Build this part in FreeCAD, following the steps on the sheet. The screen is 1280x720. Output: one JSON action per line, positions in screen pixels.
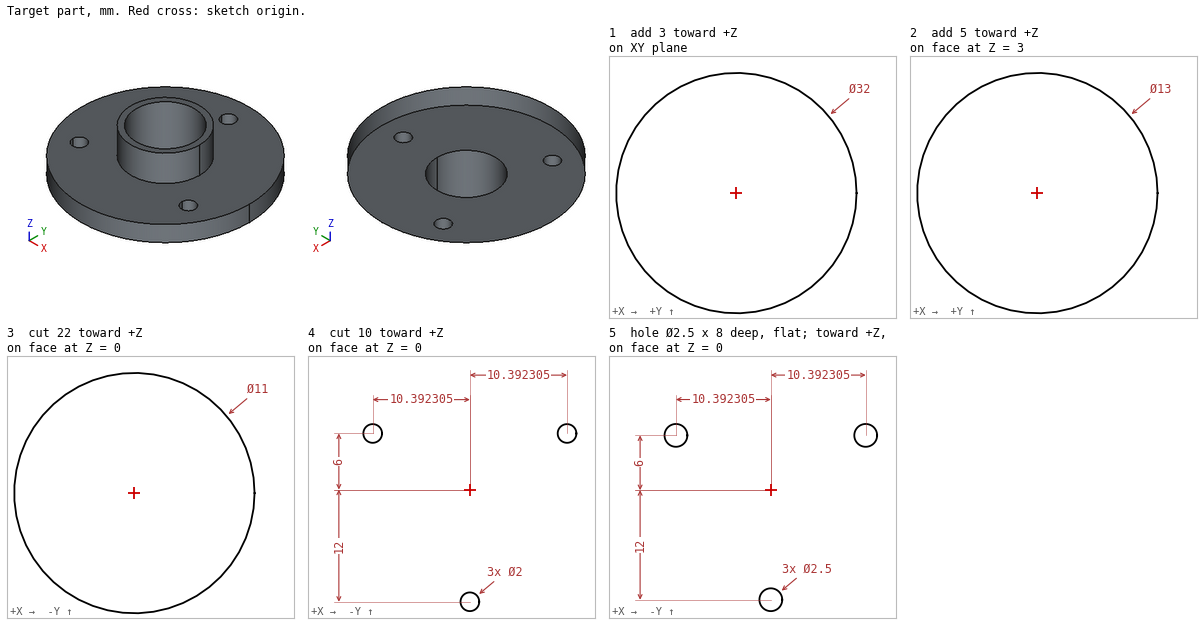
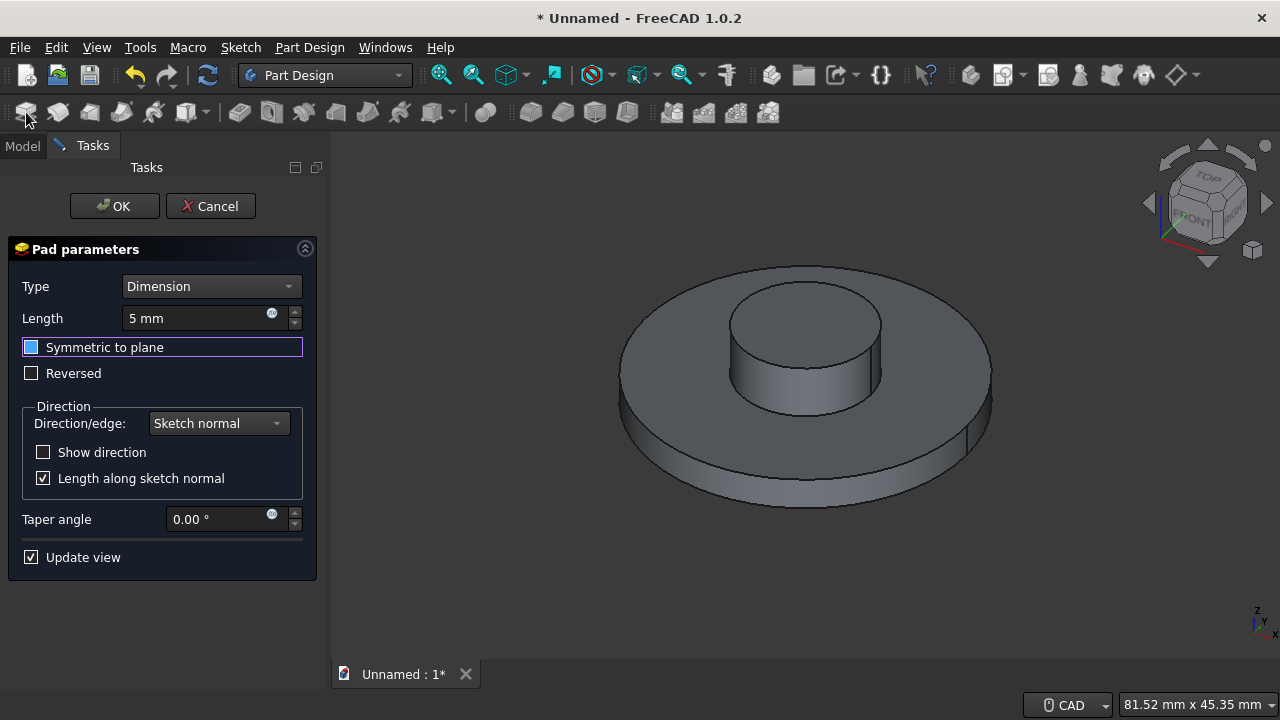
{"action": "left_click", "coordinate": [115, 206]}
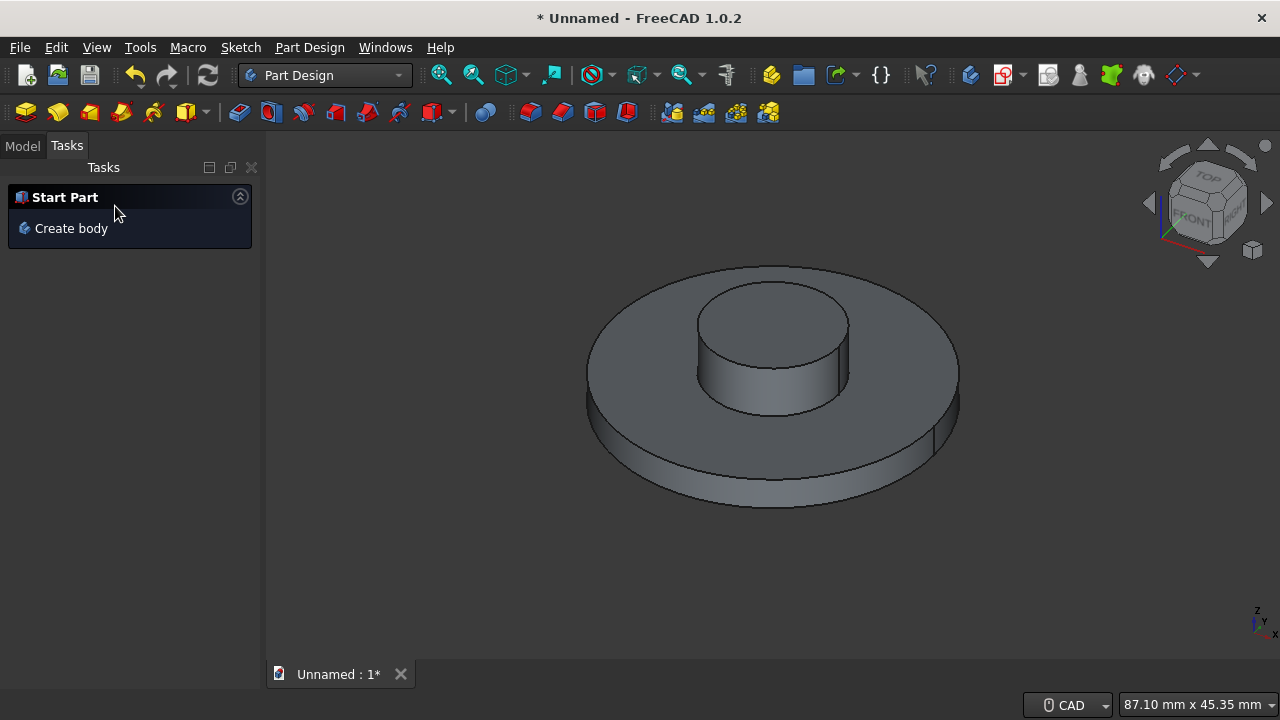
{"action": "key", "text": "5"}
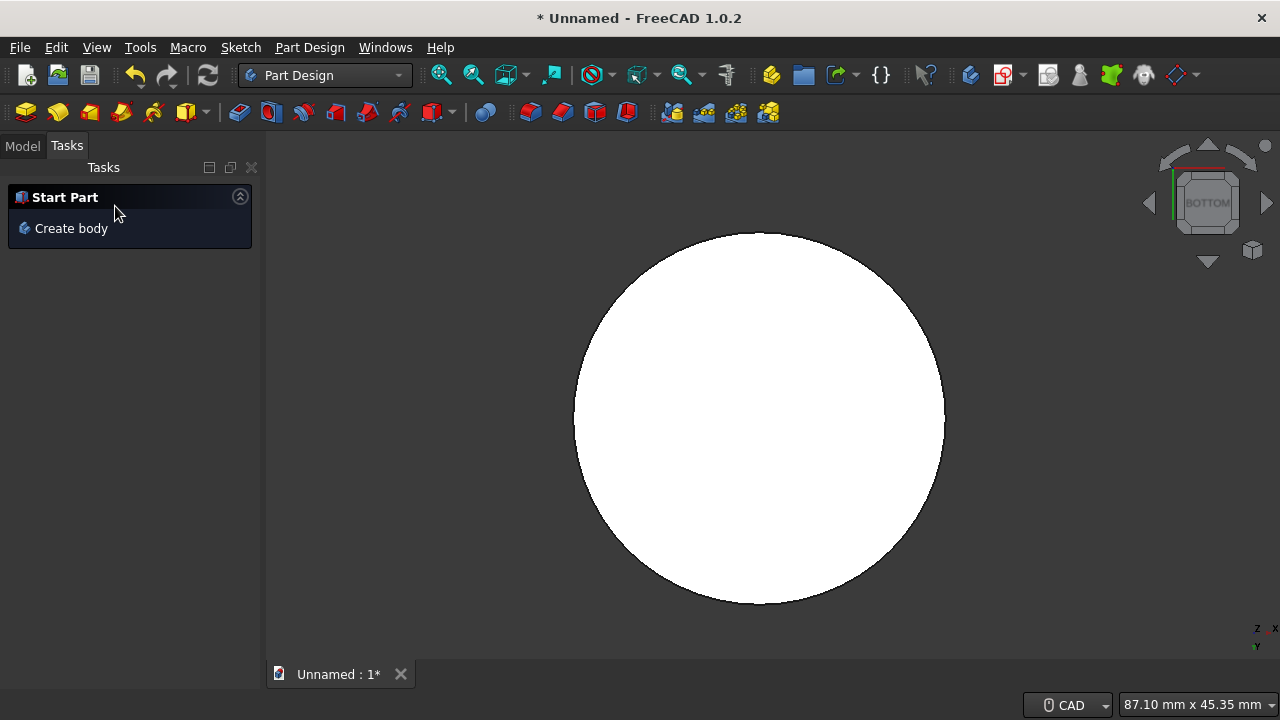
{"action": "left_click", "coordinate": [759, 418]}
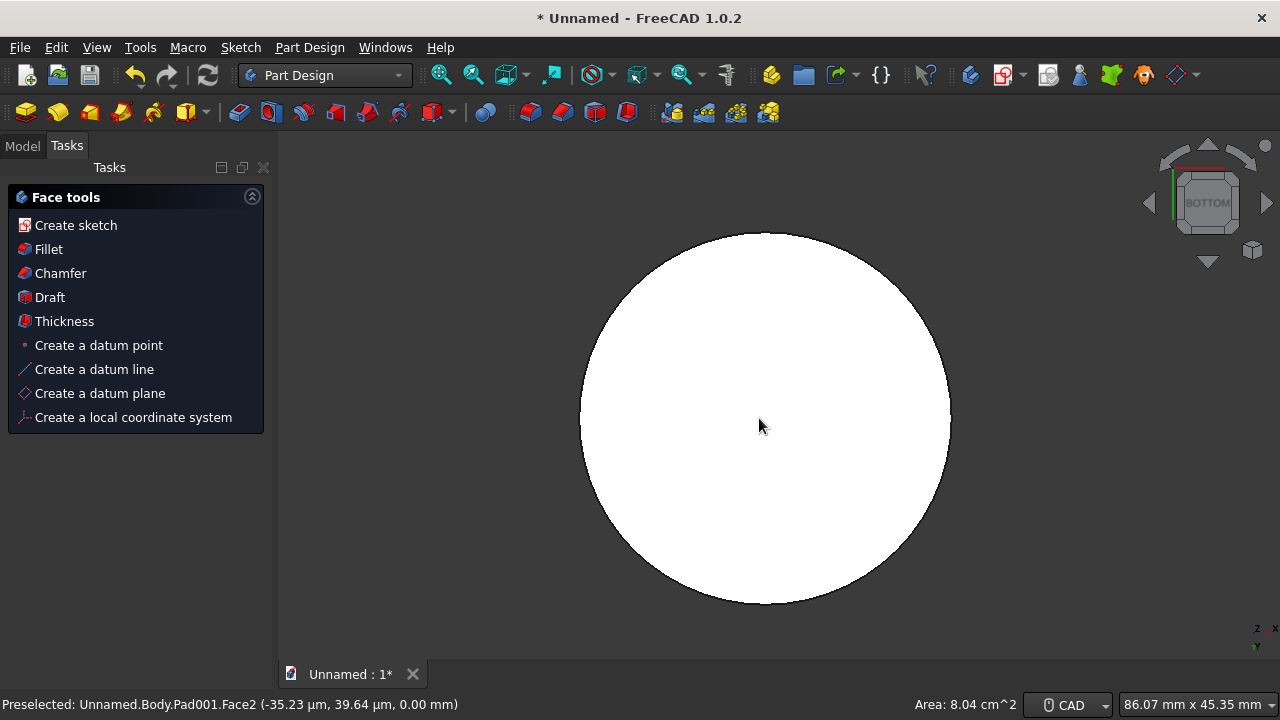
{"action": "left_click", "coordinate": [1004, 76]}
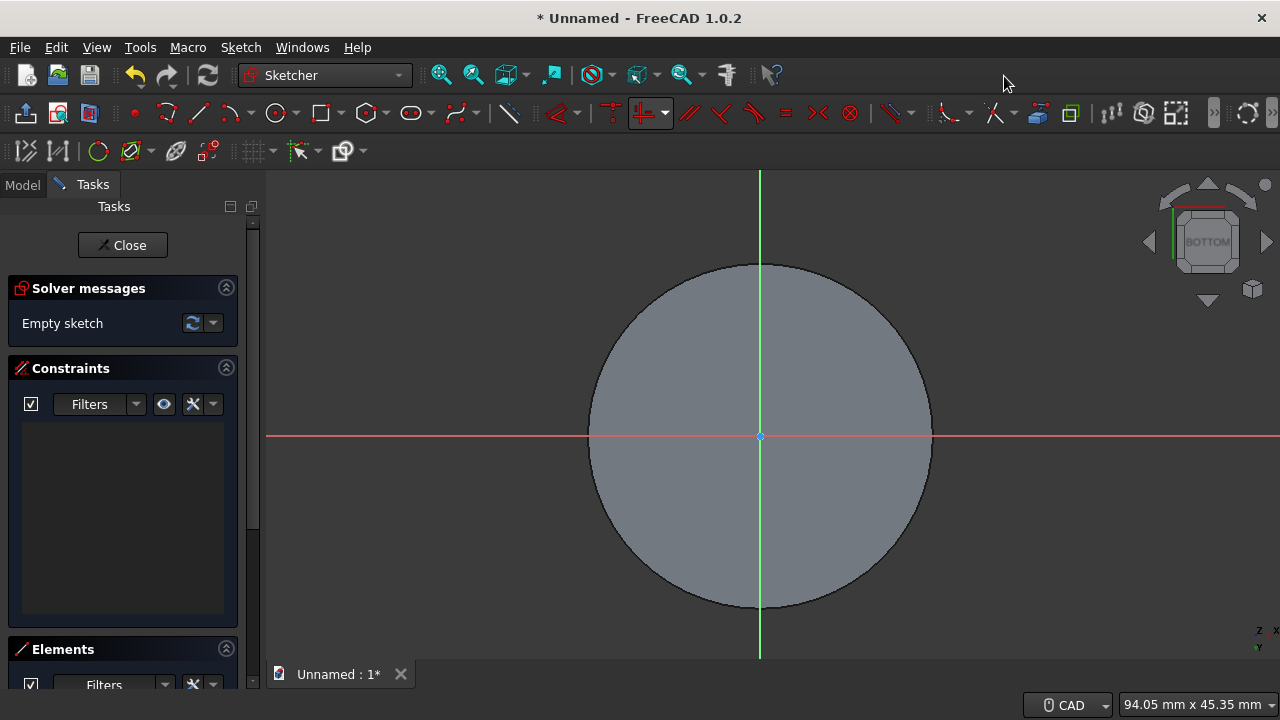
{"action": "scroll", "coordinate": [793, 449], "scroll_direction": "up", "scroll_amount": 5}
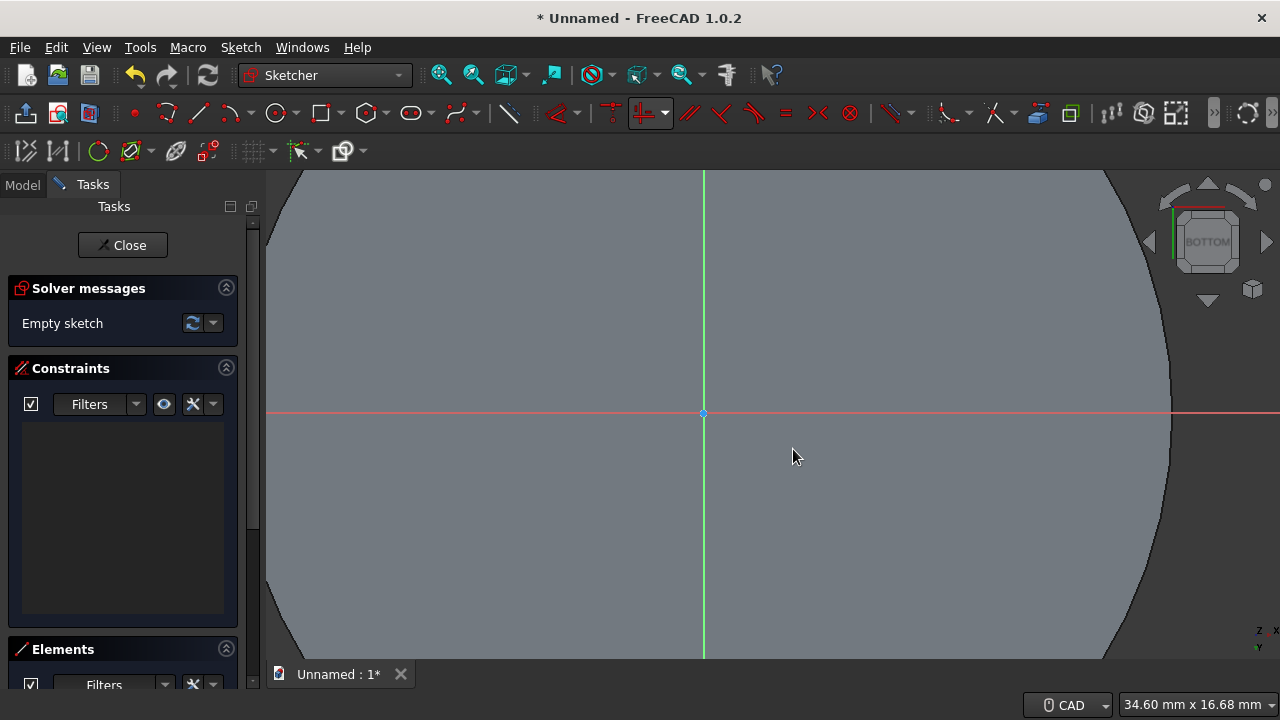
{"action": "left_click", "coordinate": [276, 114]}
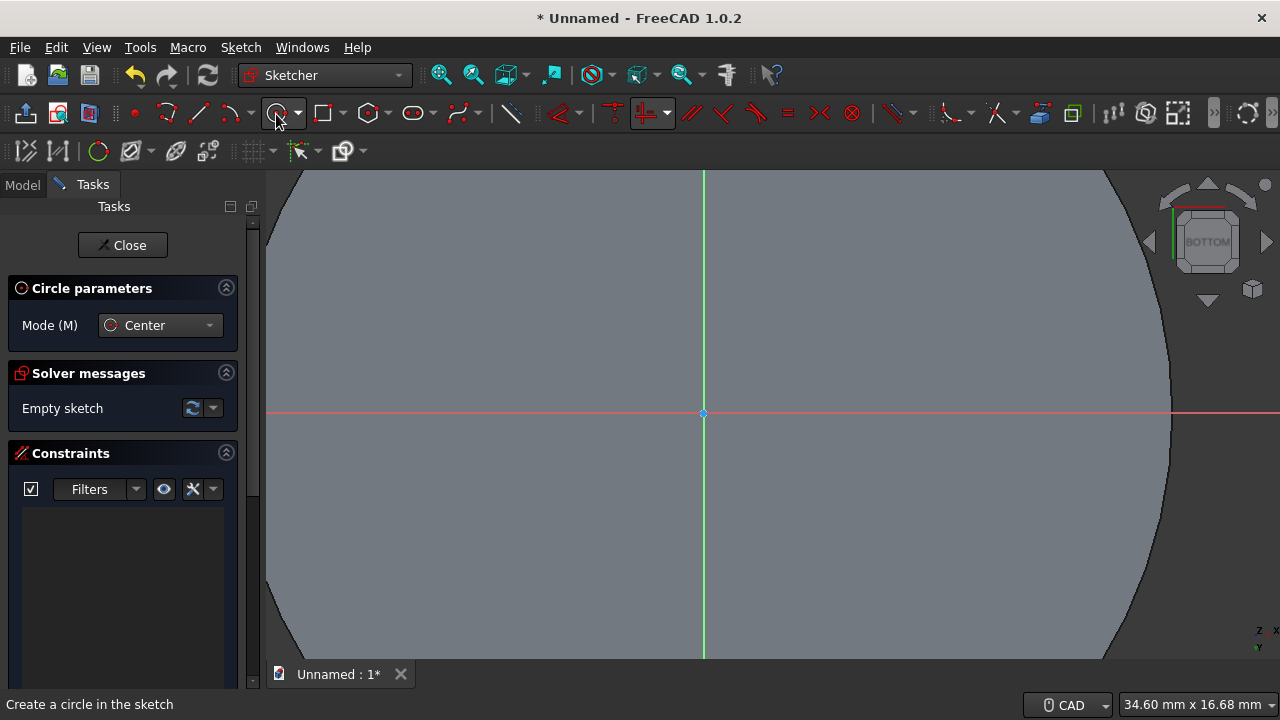
{"action": "left_click", "coordinate": [704, 413]}
{"action": "mouse_move", "coordinate": [818, 300]}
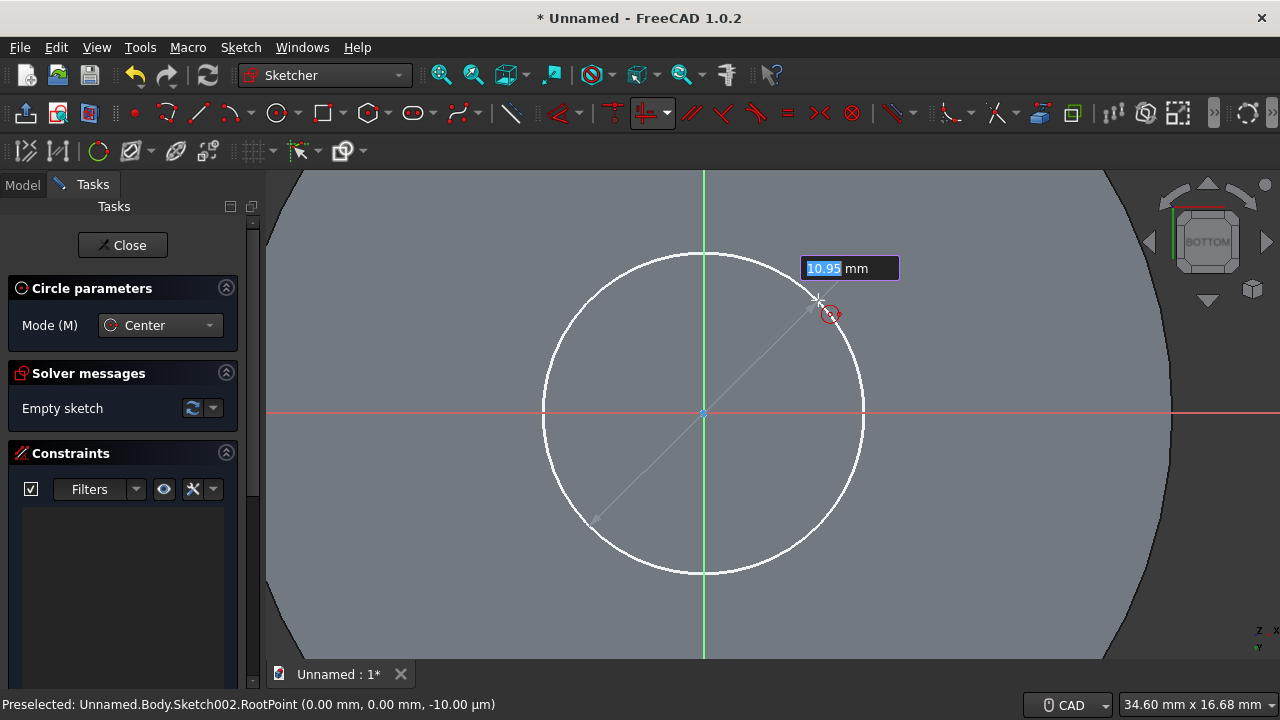
{"action": "type", "text": "11"}
{"action": "key", "text": "Return"}
{"action": "key", "text": "Escape"}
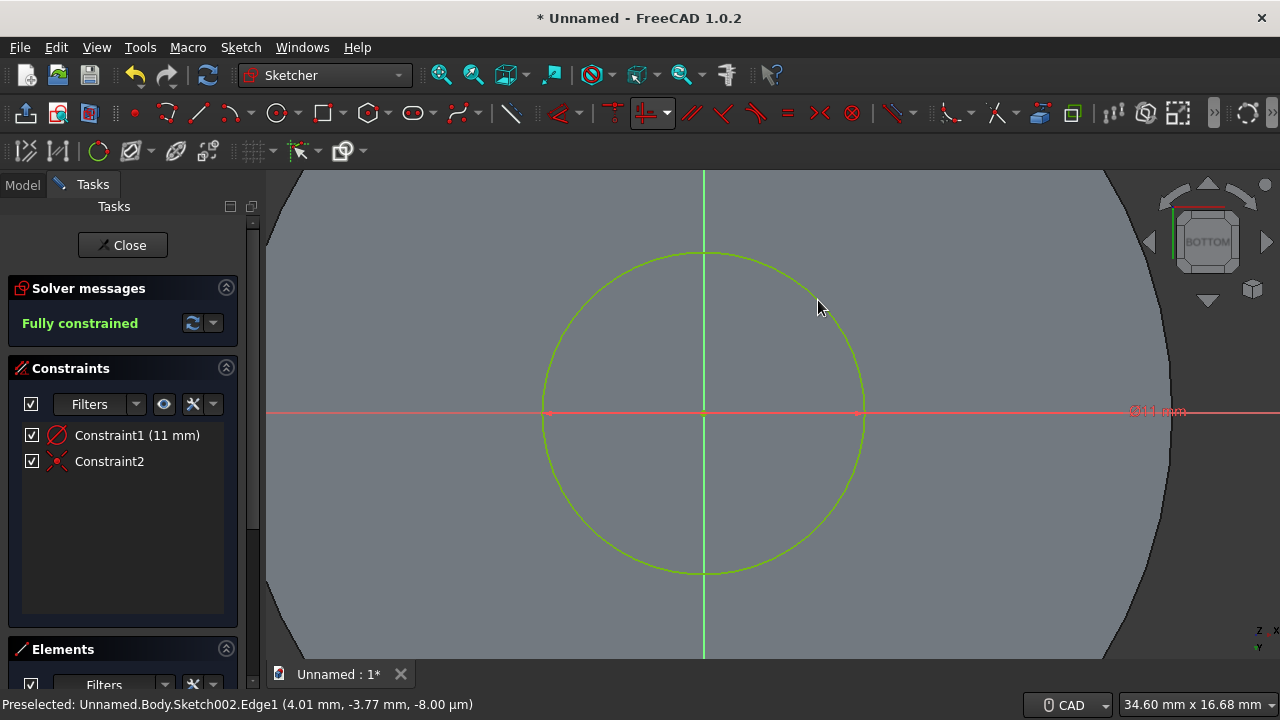
{"action": "left_click", "coordinate": [123, 245]}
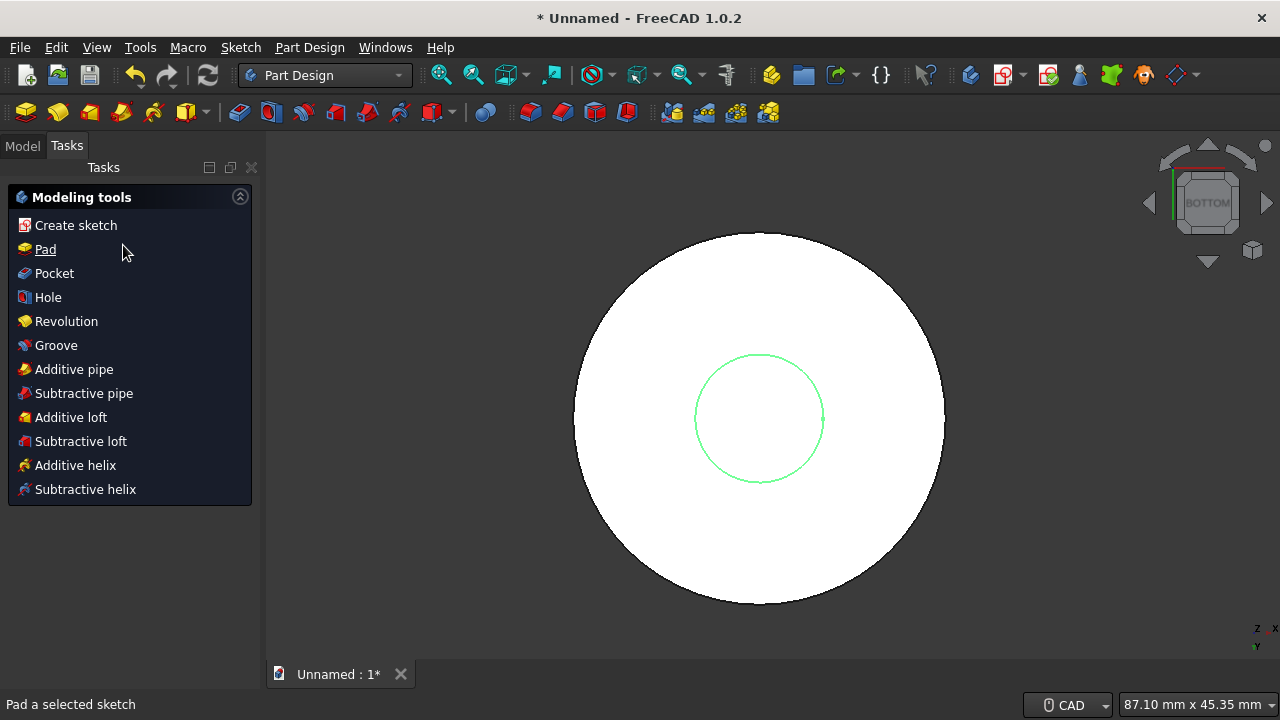
{"action": "left_click", "coordinate": [240, 112]}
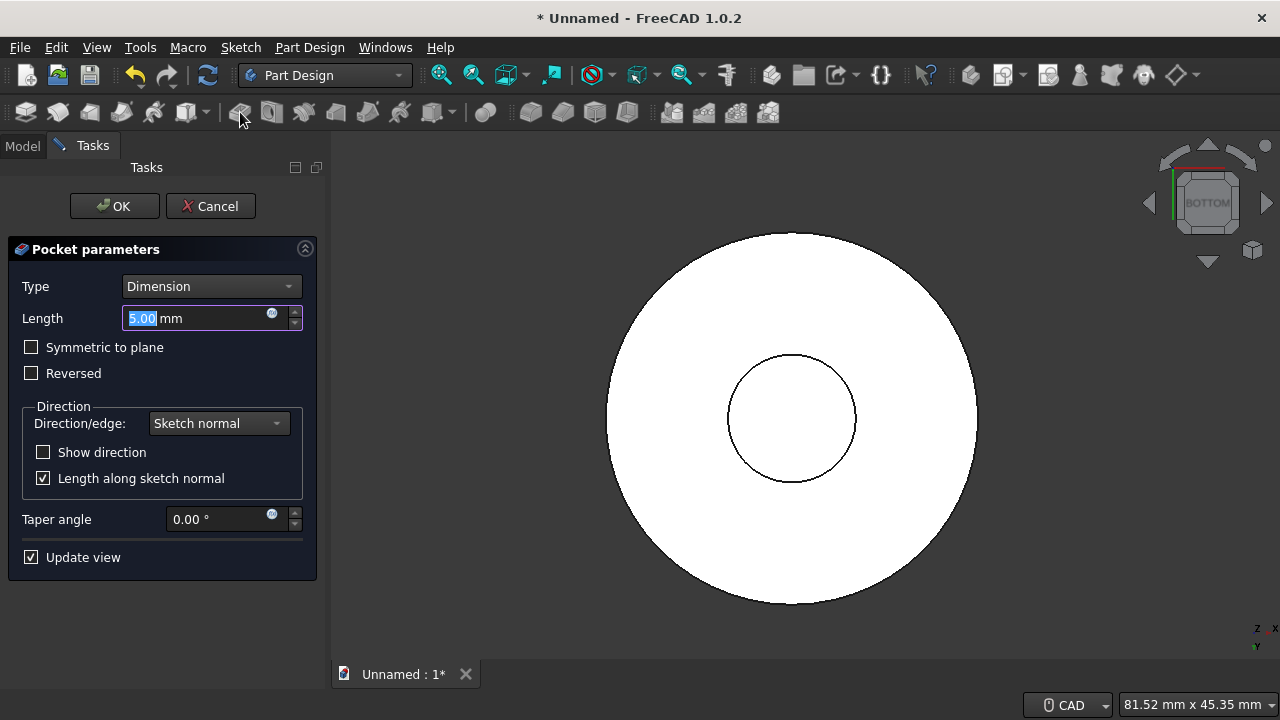
{"action": "type", "text": "22"}
{"action": "key", "text": "Tab"}